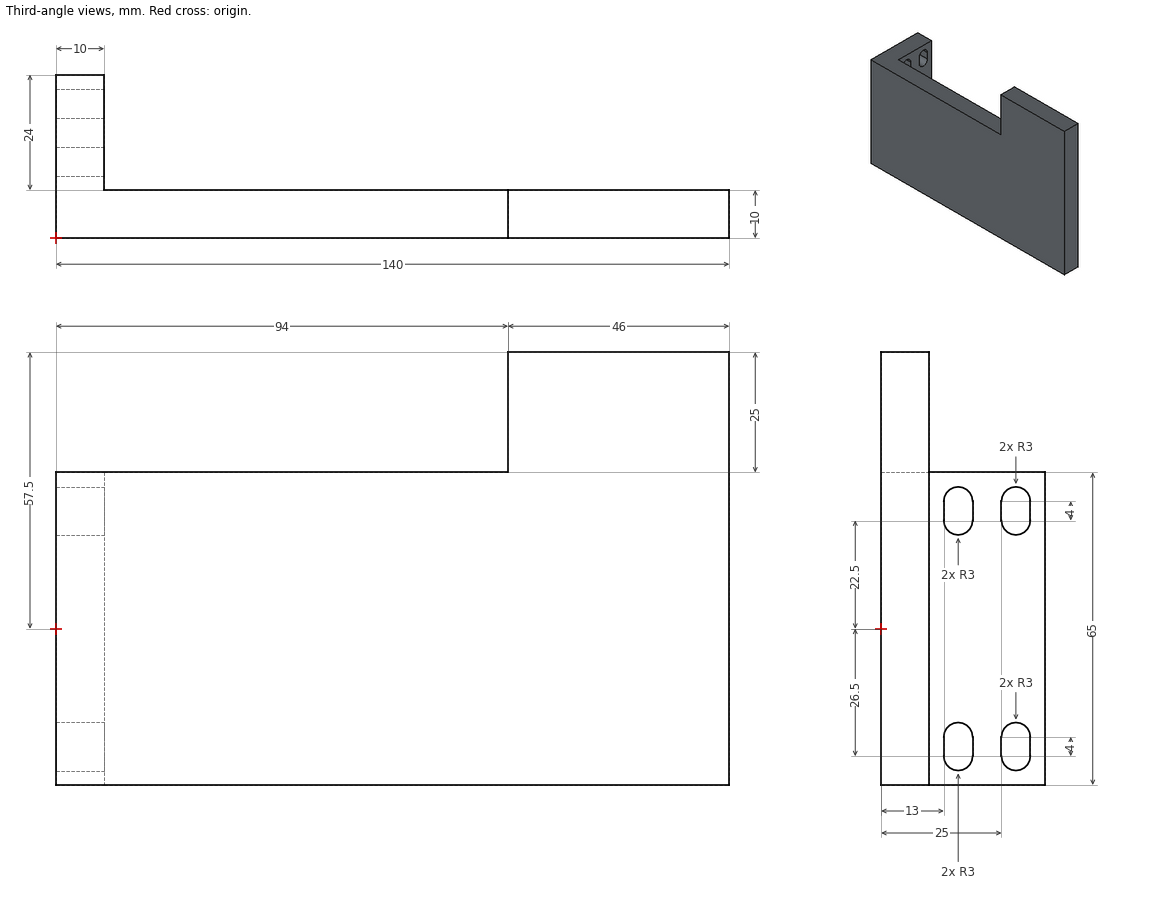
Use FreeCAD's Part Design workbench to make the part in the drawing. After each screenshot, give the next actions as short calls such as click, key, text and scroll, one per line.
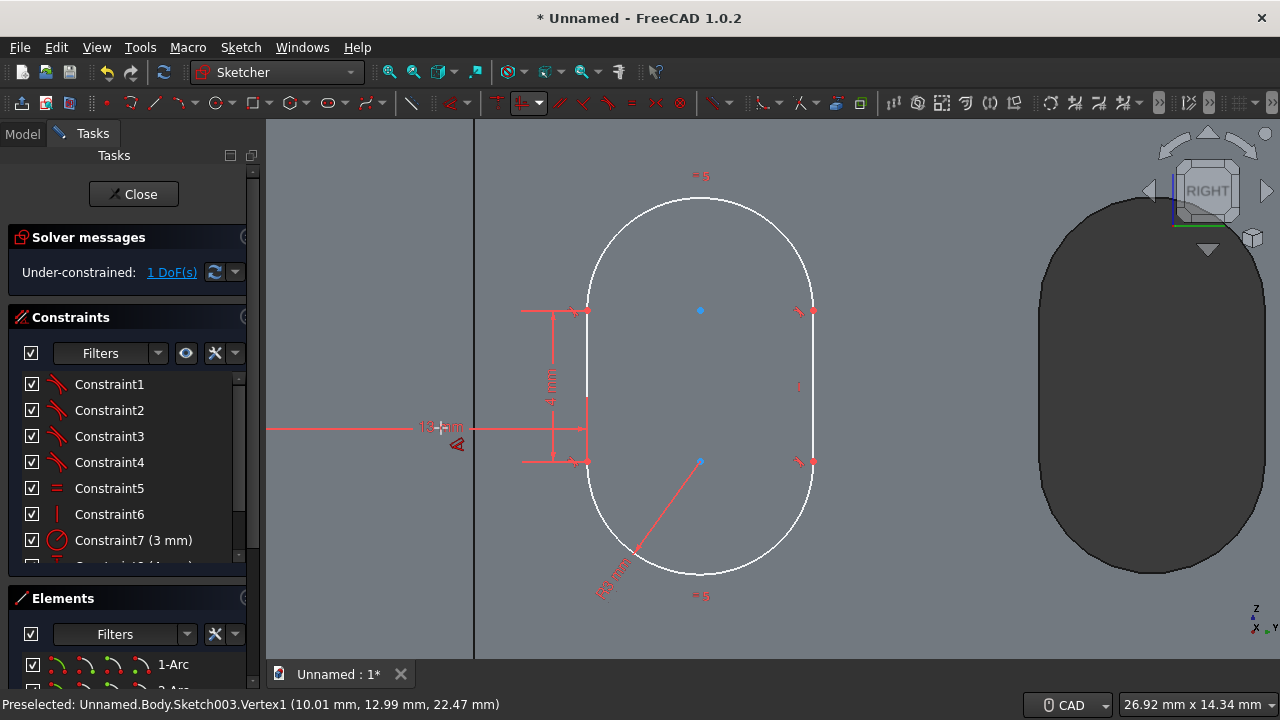
click(587, 462)
click(621, 507)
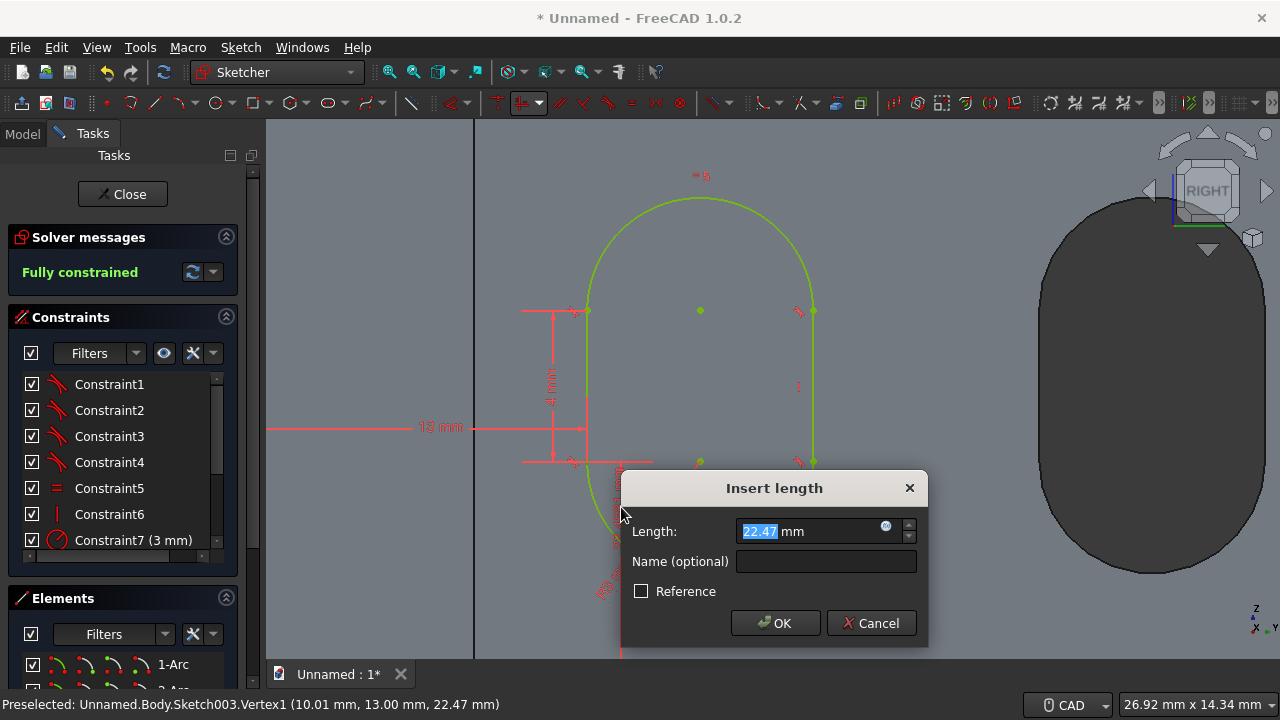
text(22.5)
key(Return)
key(Escape)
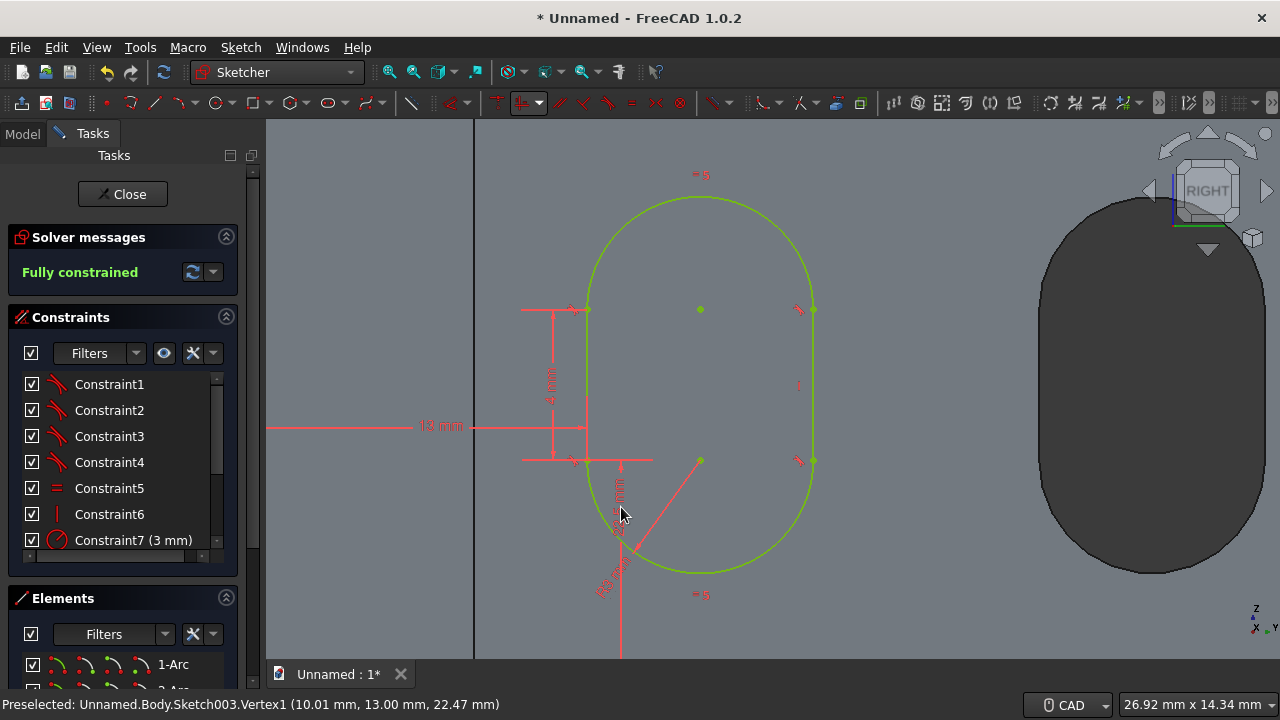
click(123, 194)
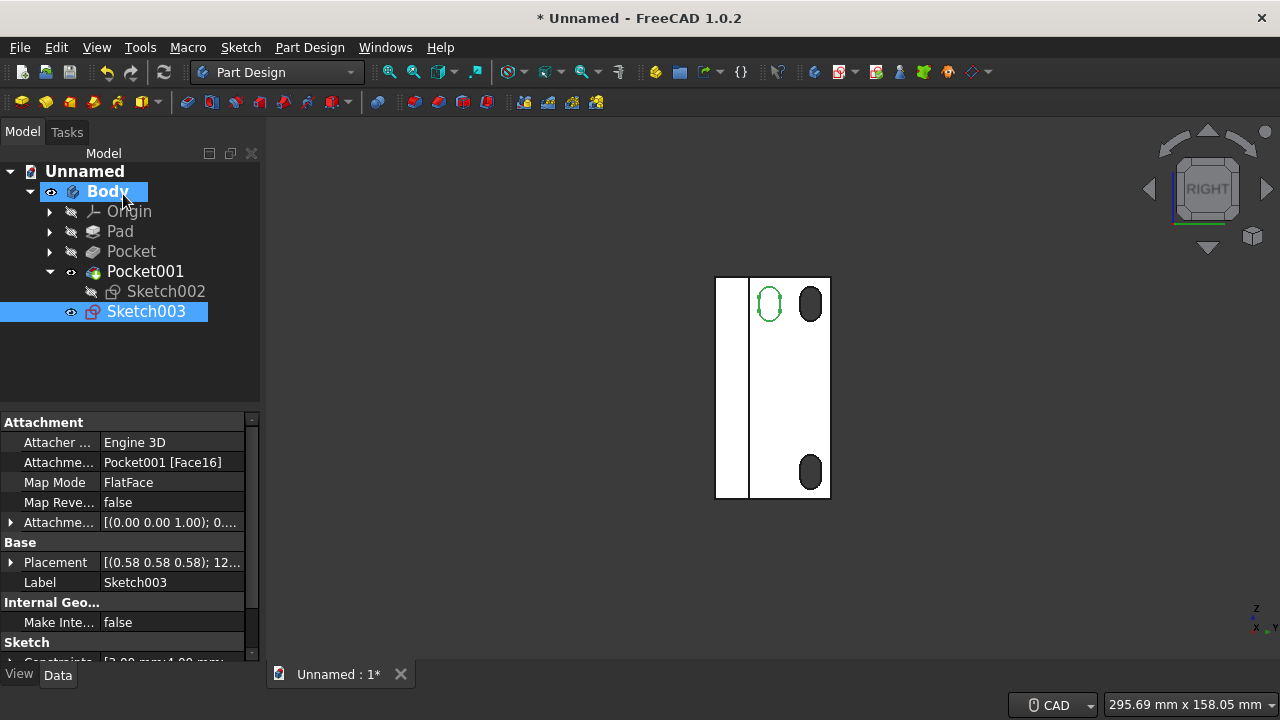
click(188, 102)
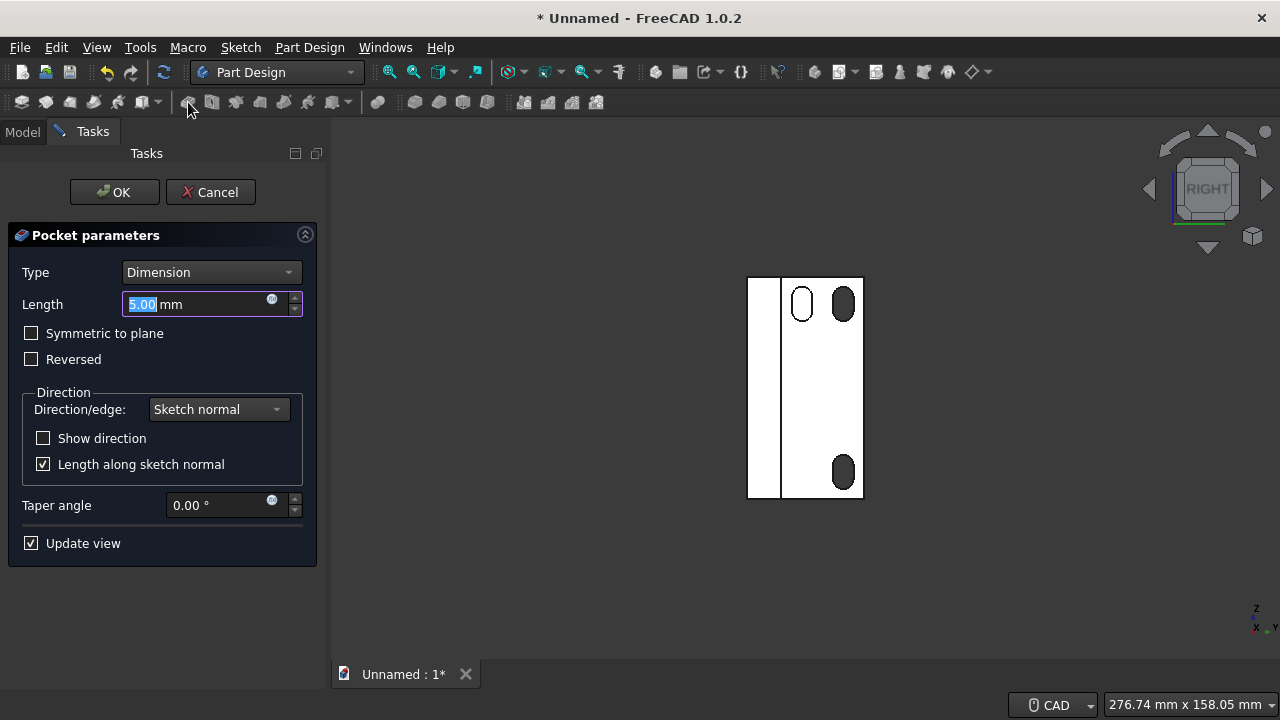
click(212, 272)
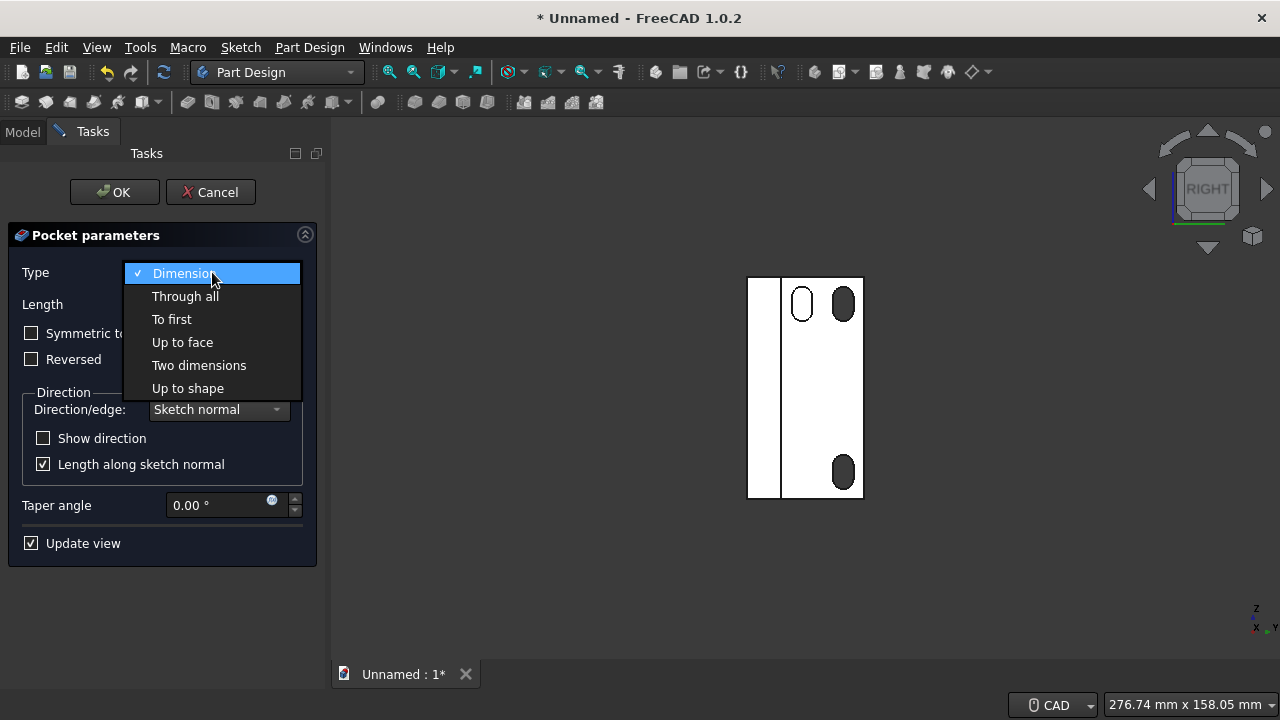
click(212, 320)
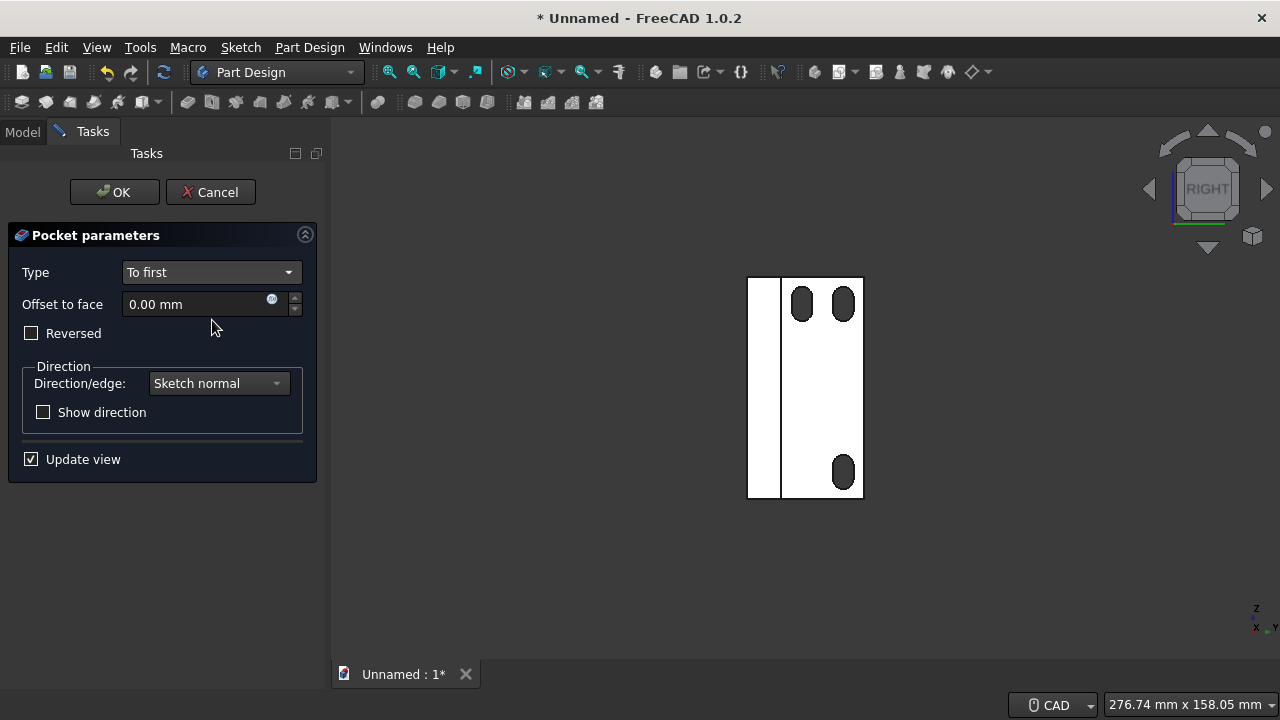
click(115, 192)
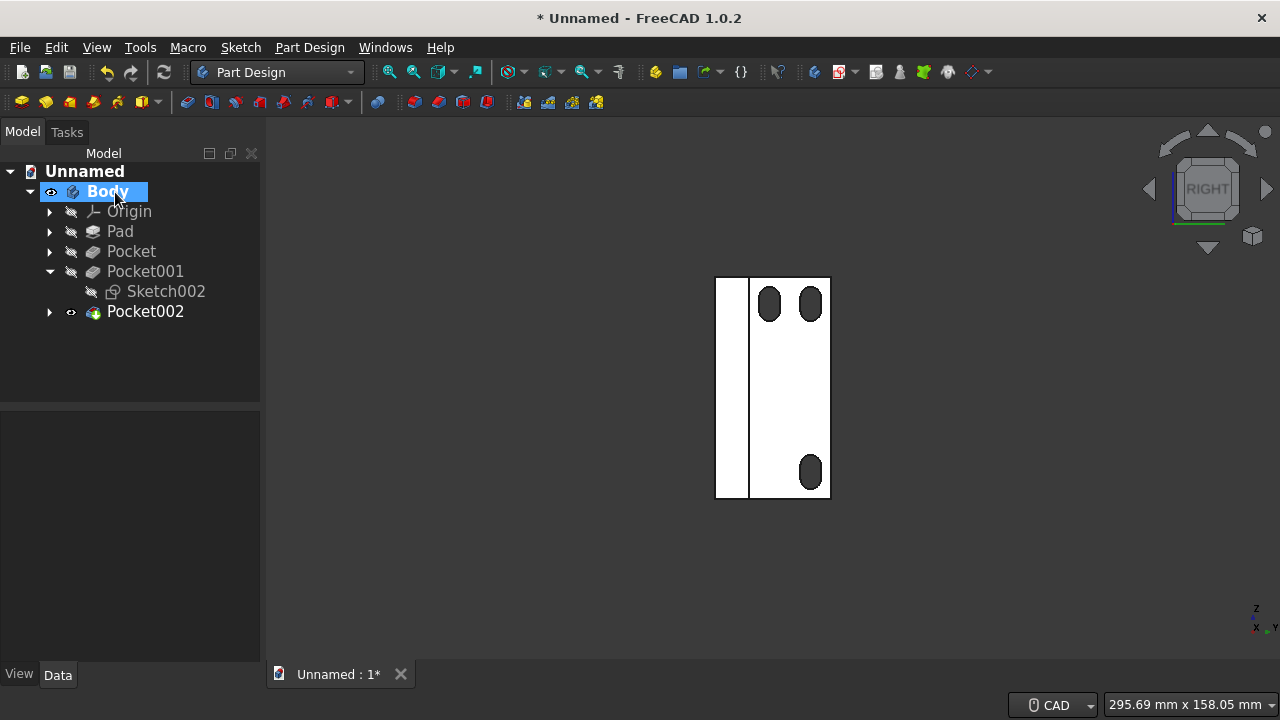
key(v)
key(f)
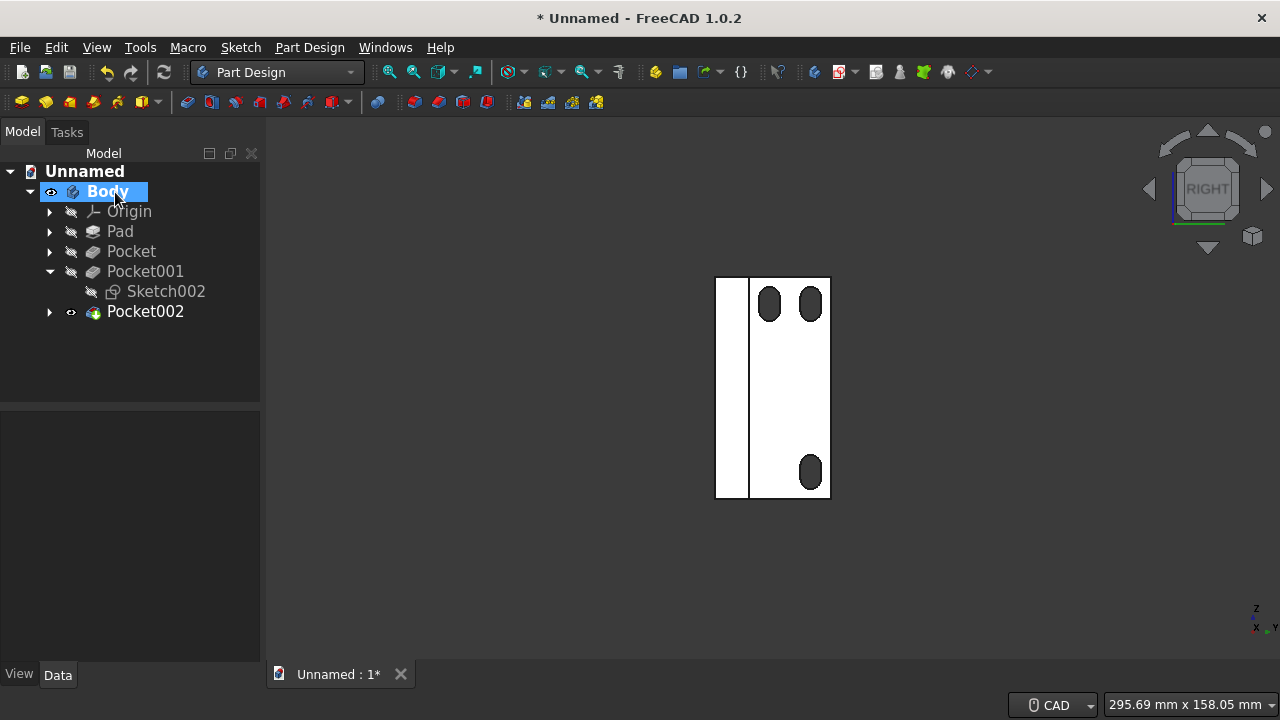
click(790, 387)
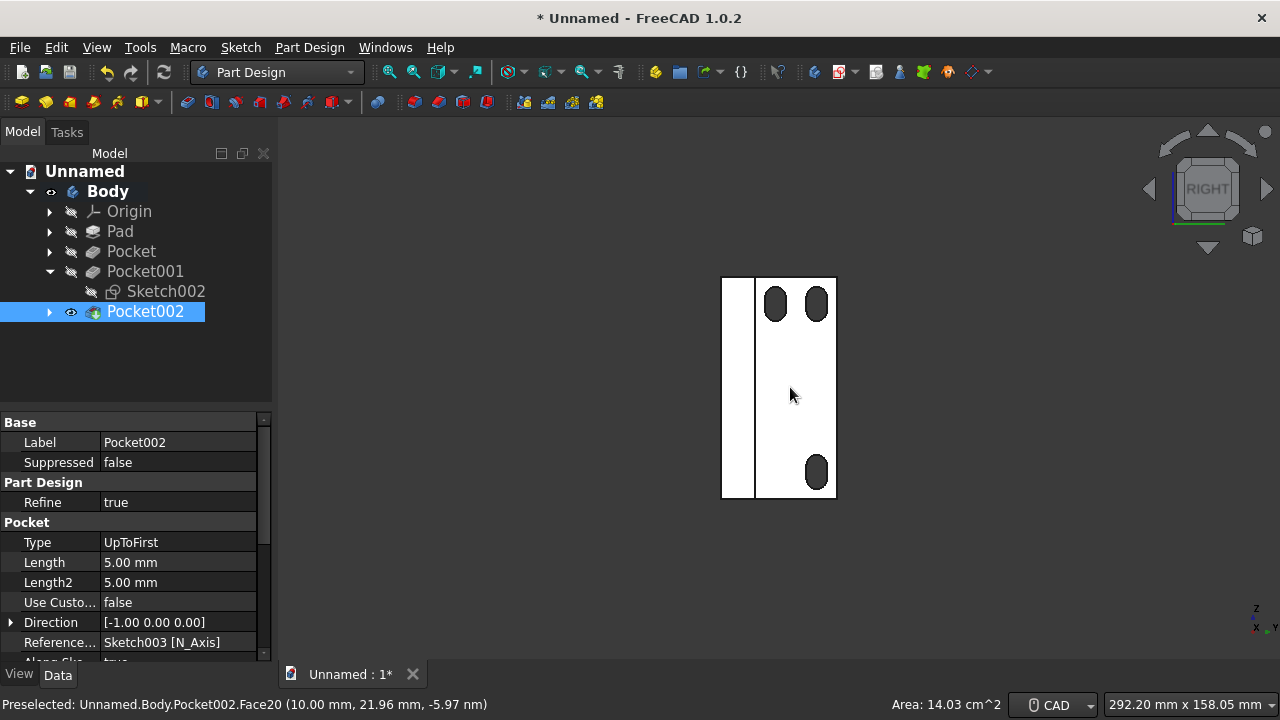
click(840, 72)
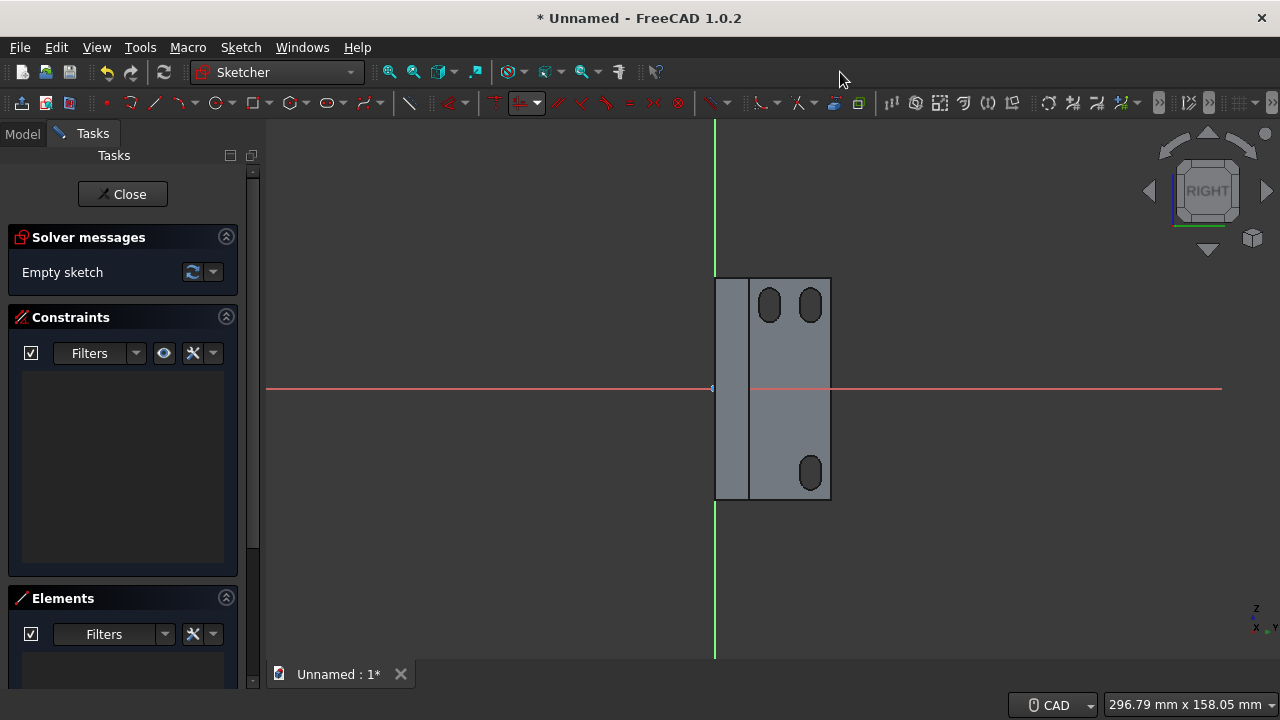
key(q)
key(s)